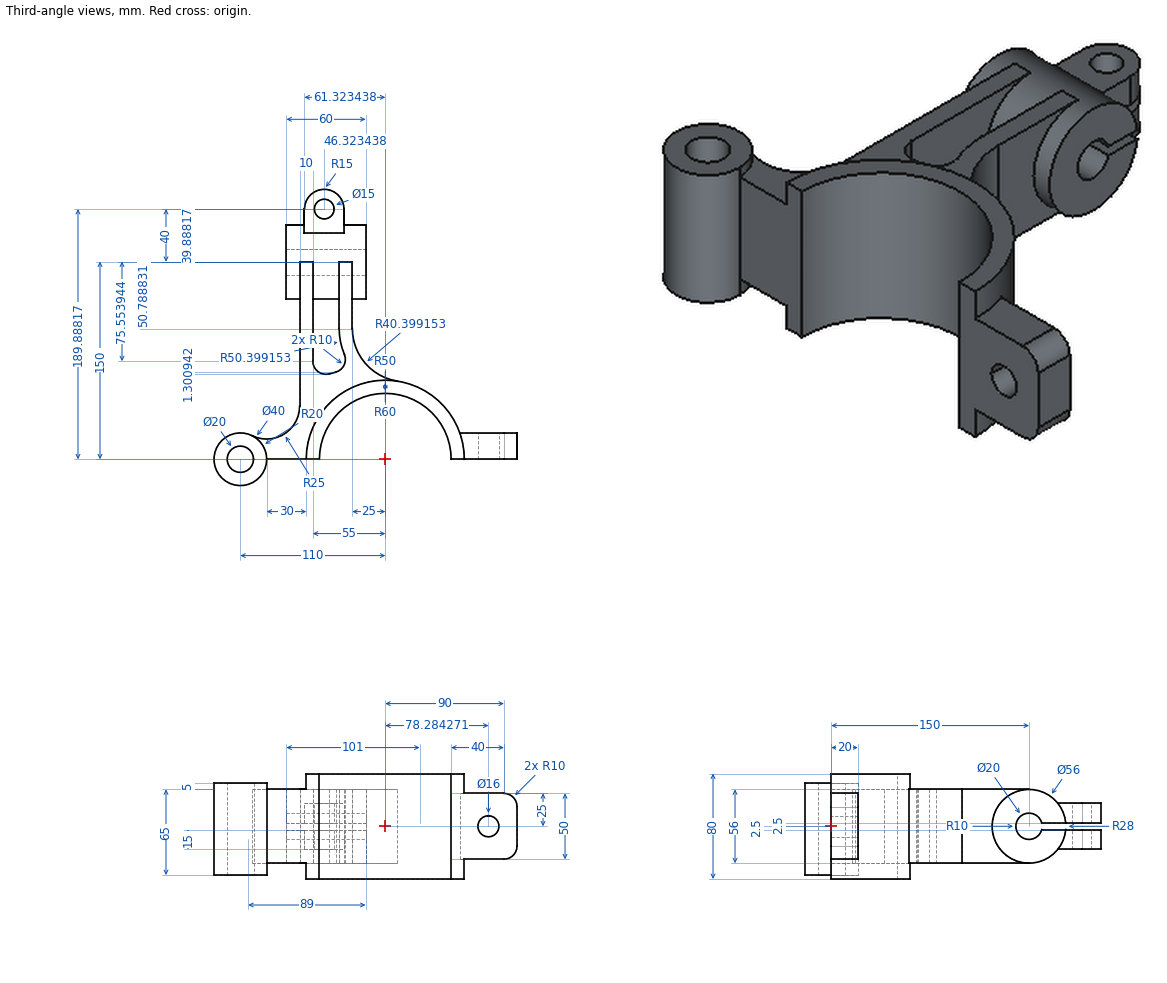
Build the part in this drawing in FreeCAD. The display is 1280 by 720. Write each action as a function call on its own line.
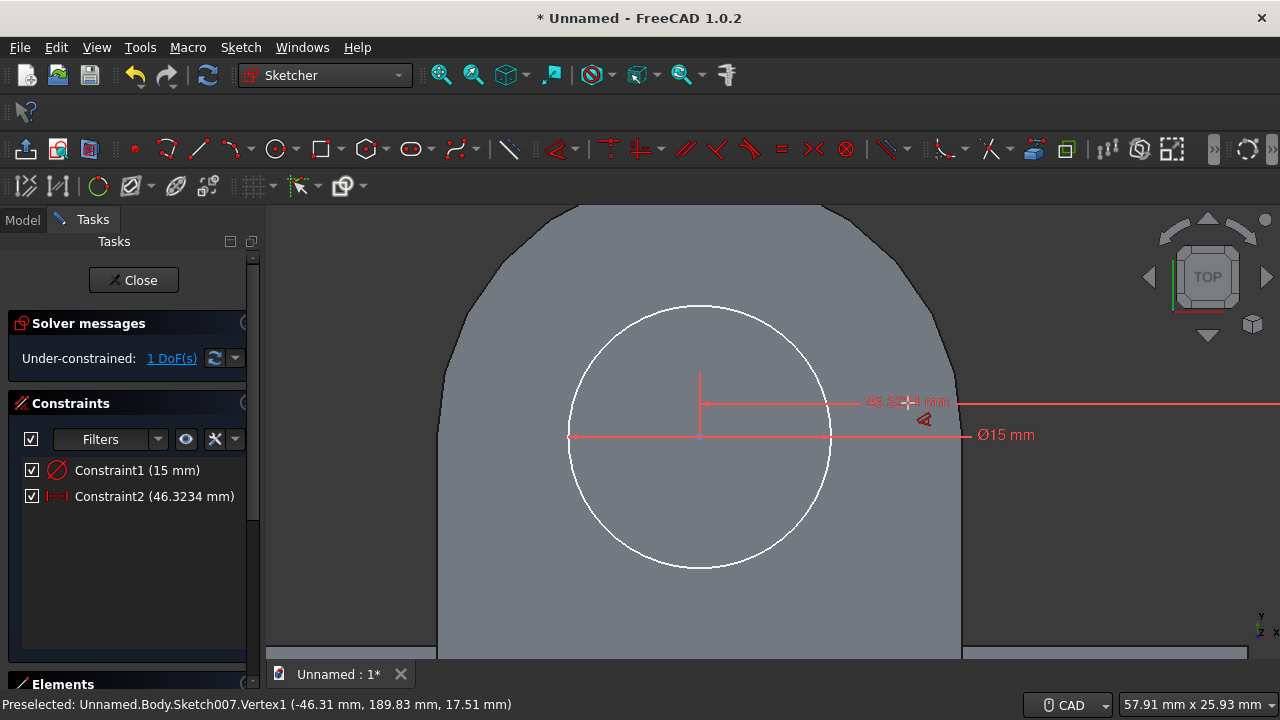
click(700, 437)
click(666, 534)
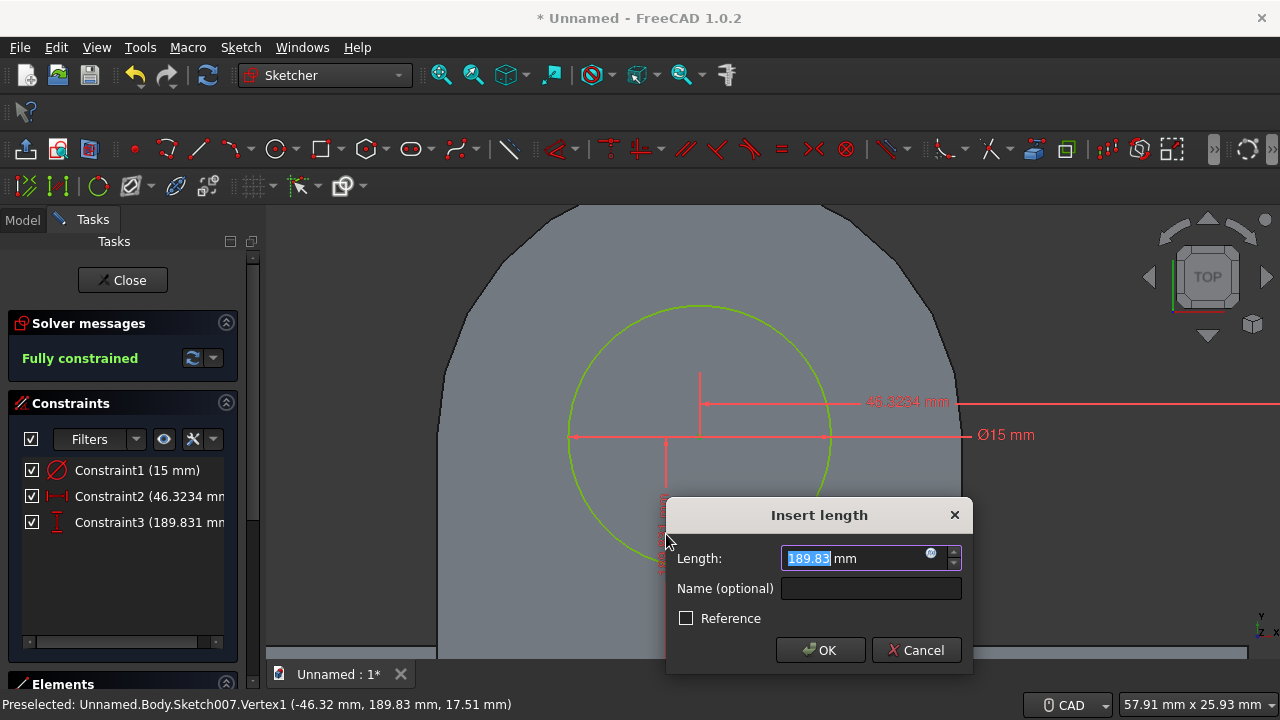
text(189.88817)
key(Return)
key(Escape)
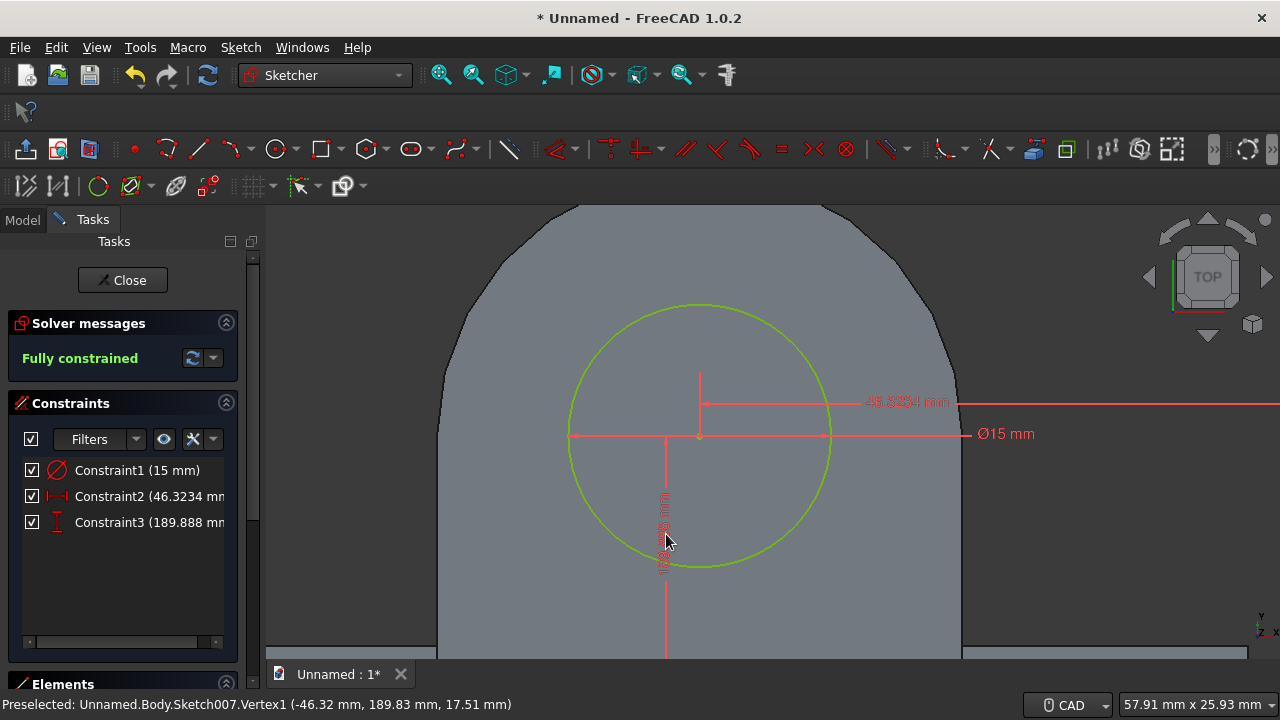
click(123, 280)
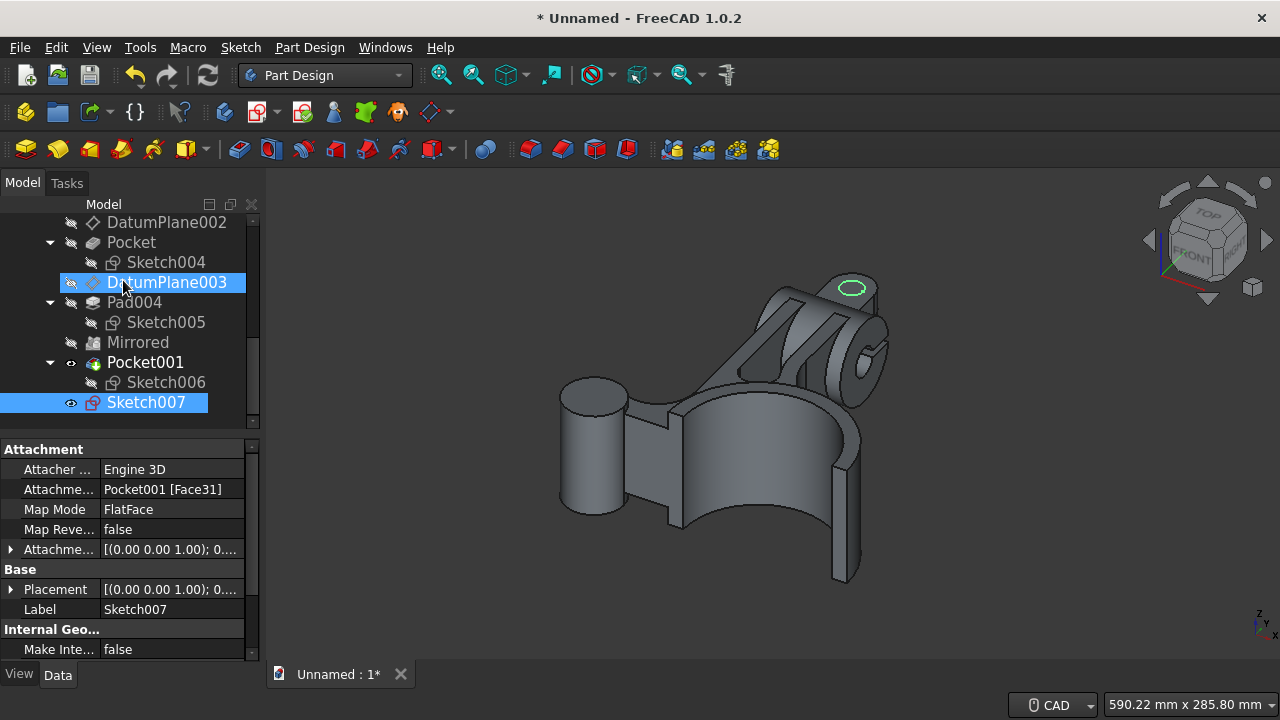
click(240, 150)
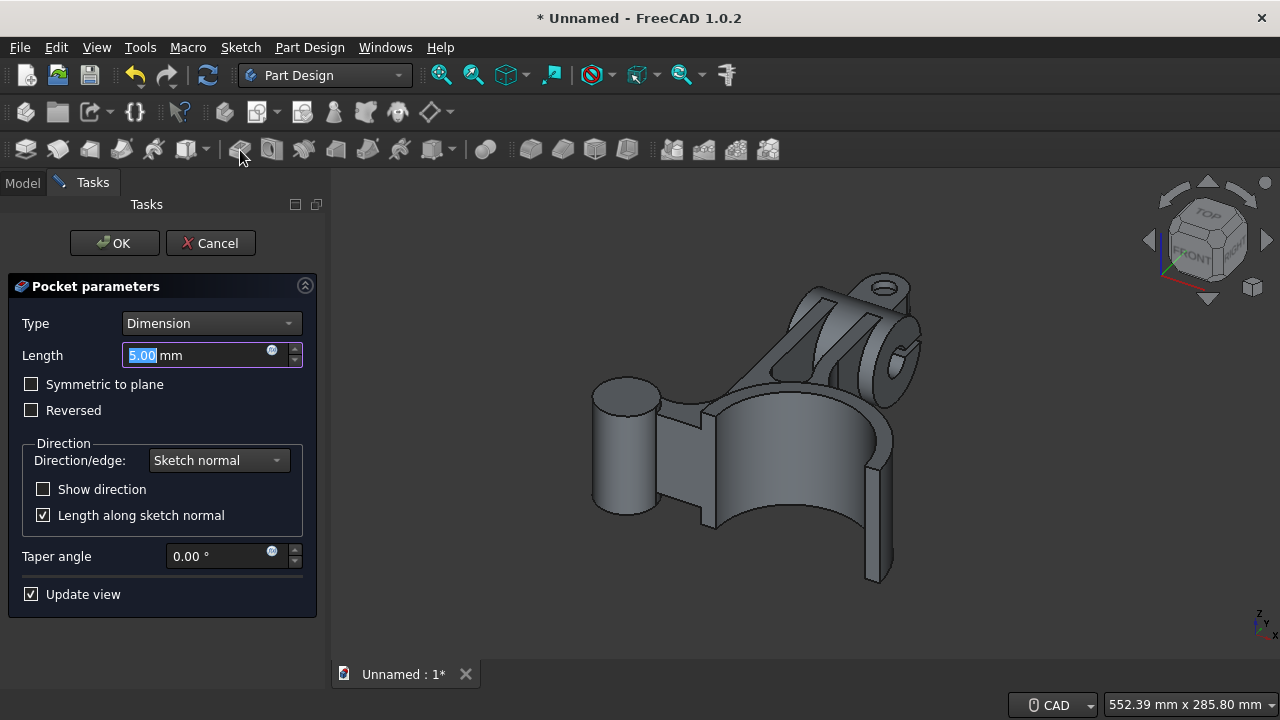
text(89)
key(Tab)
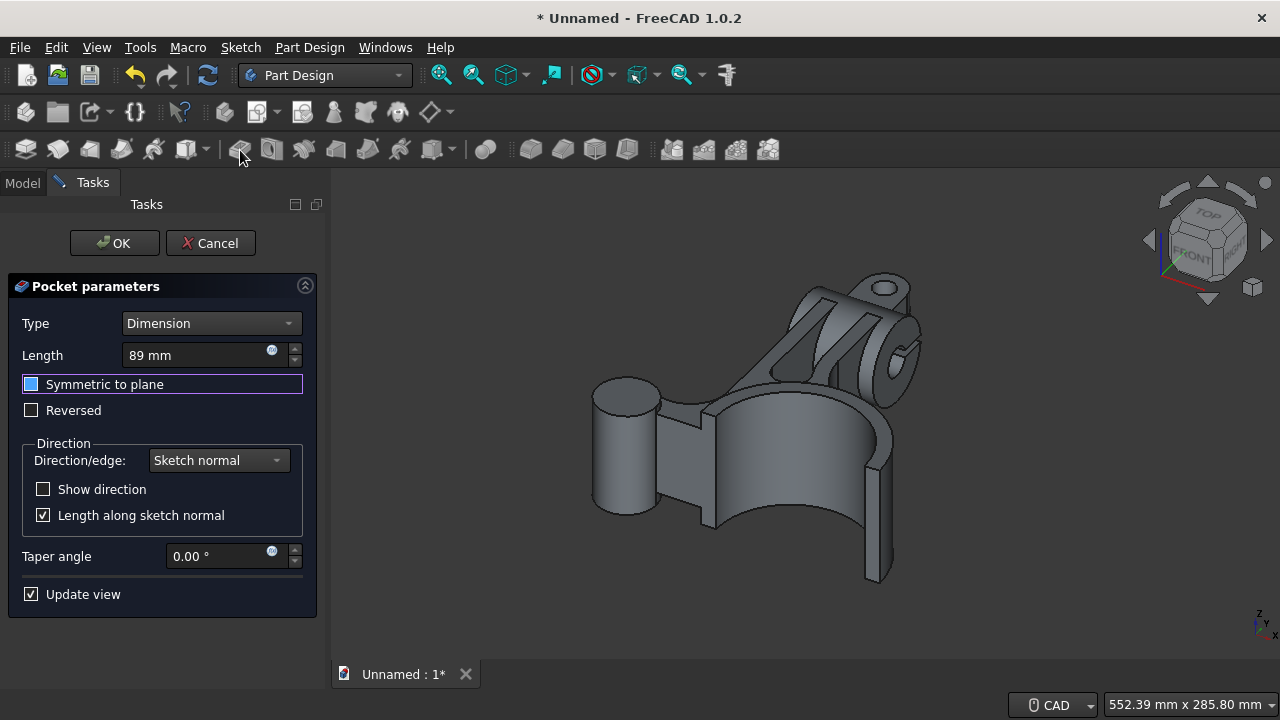
click(115, 243)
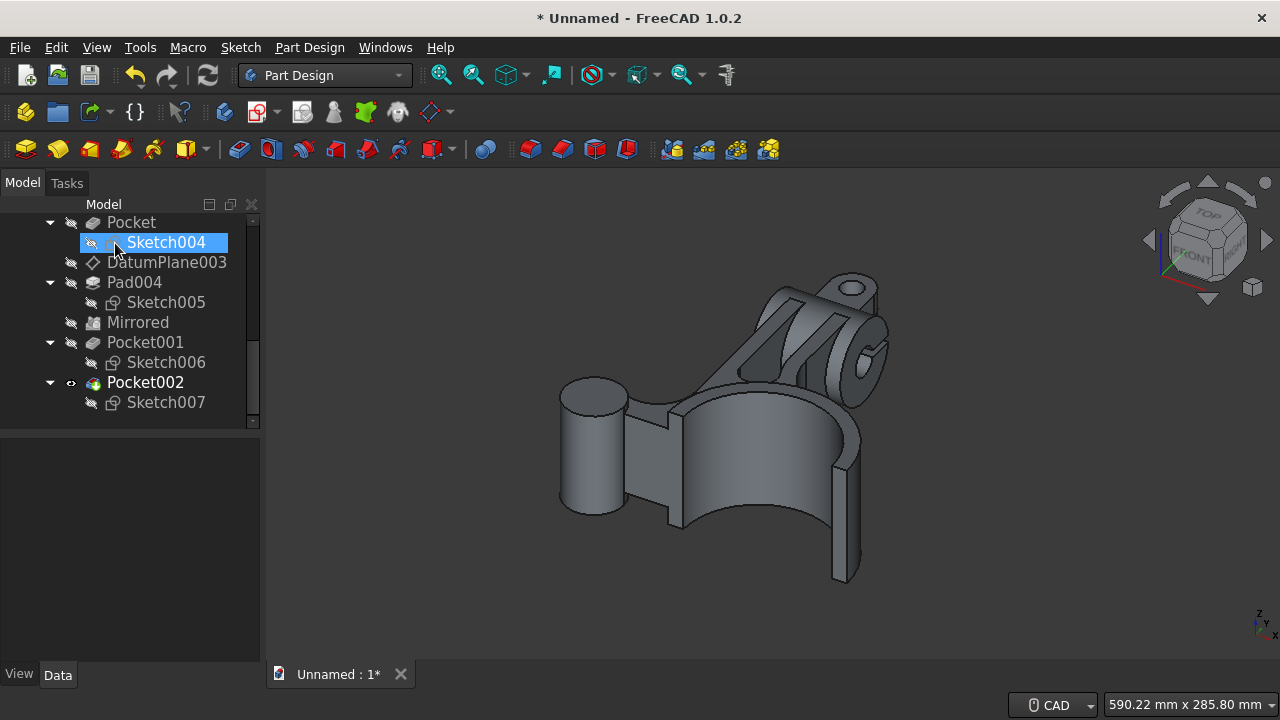
click(594, 396)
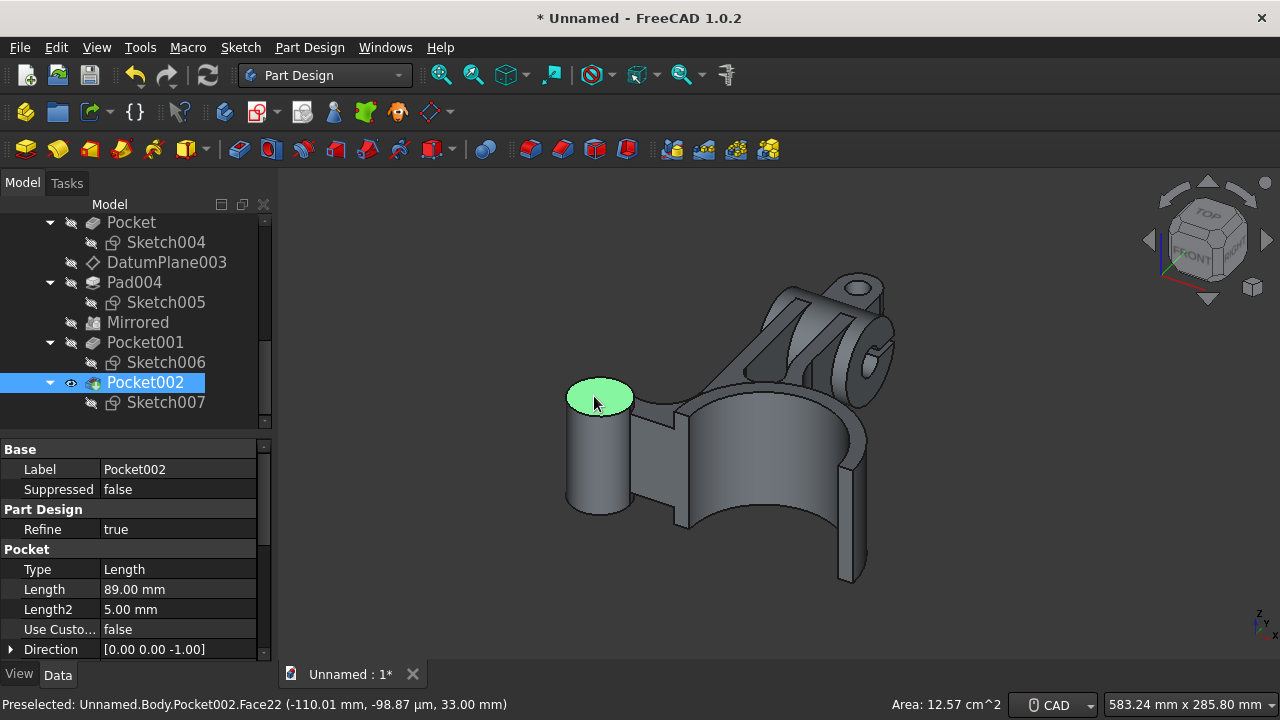
click(258, 112)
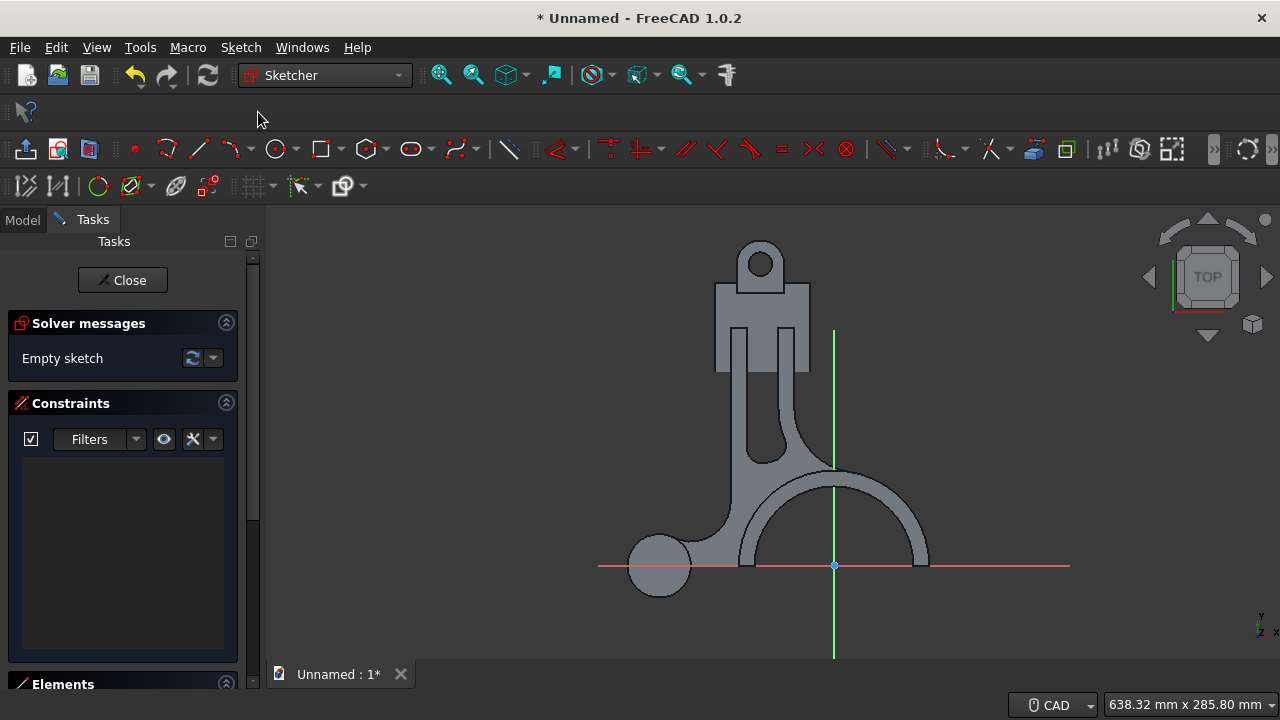
scroll(654, 583, up, 11)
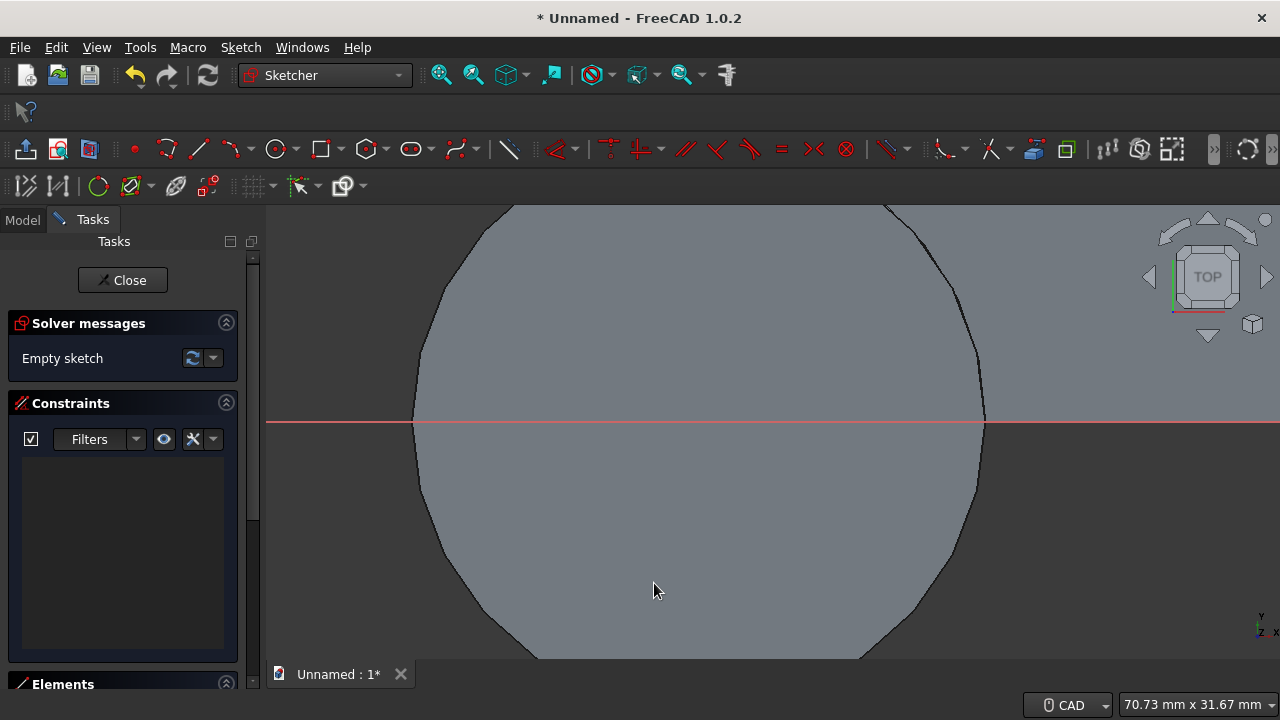
key(g)
key(c)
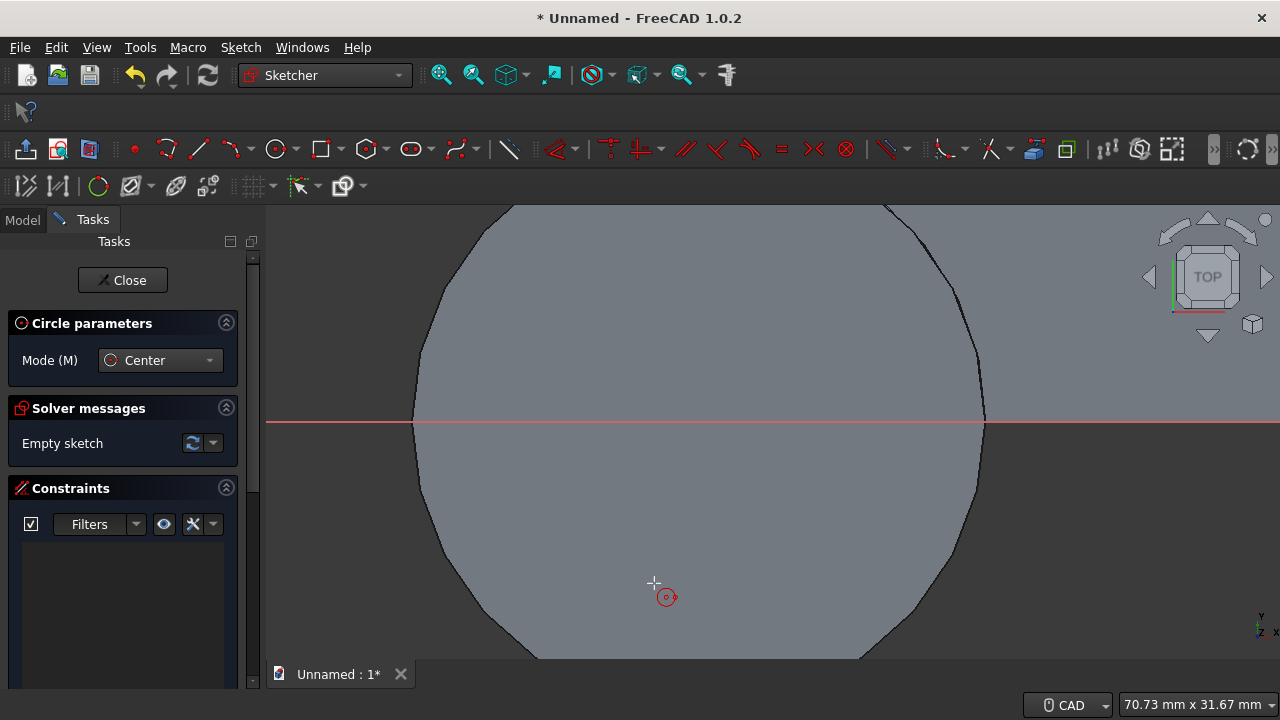
click(699, 422)
move(800, 320)